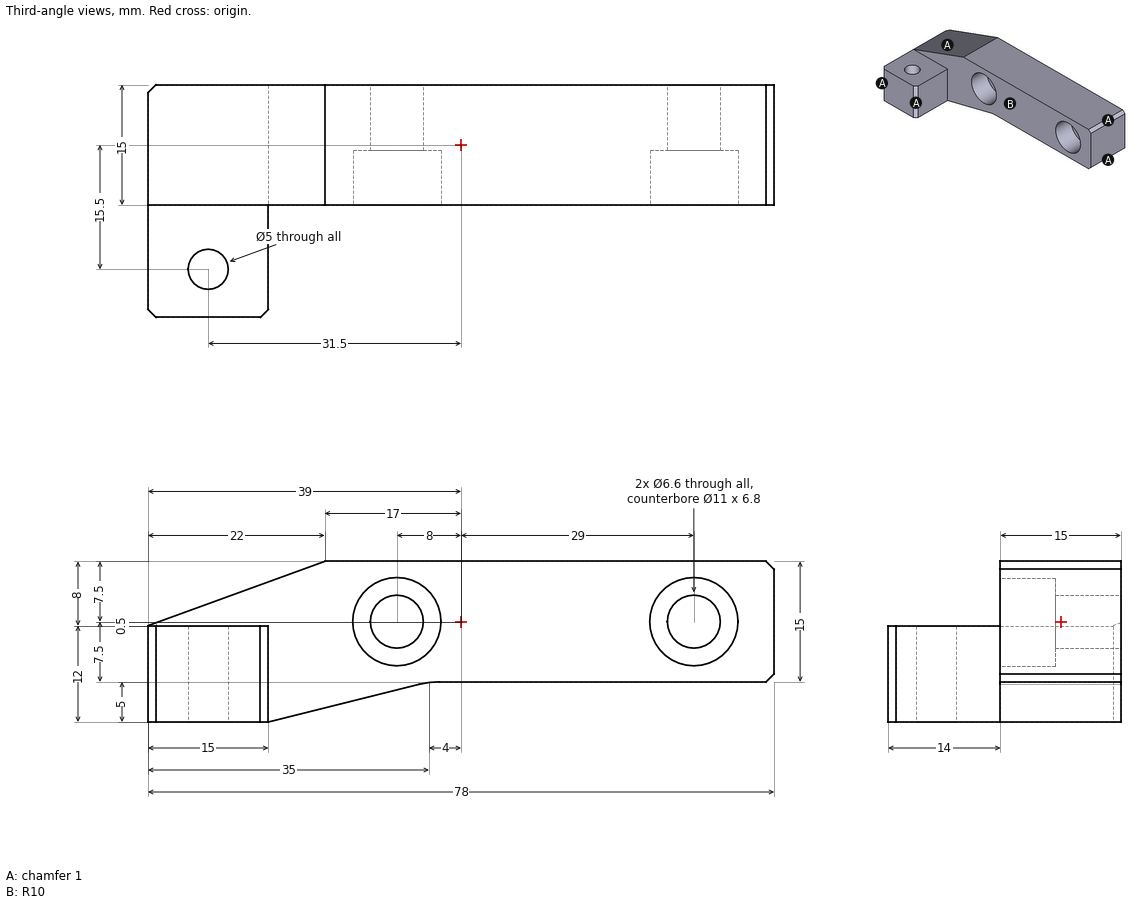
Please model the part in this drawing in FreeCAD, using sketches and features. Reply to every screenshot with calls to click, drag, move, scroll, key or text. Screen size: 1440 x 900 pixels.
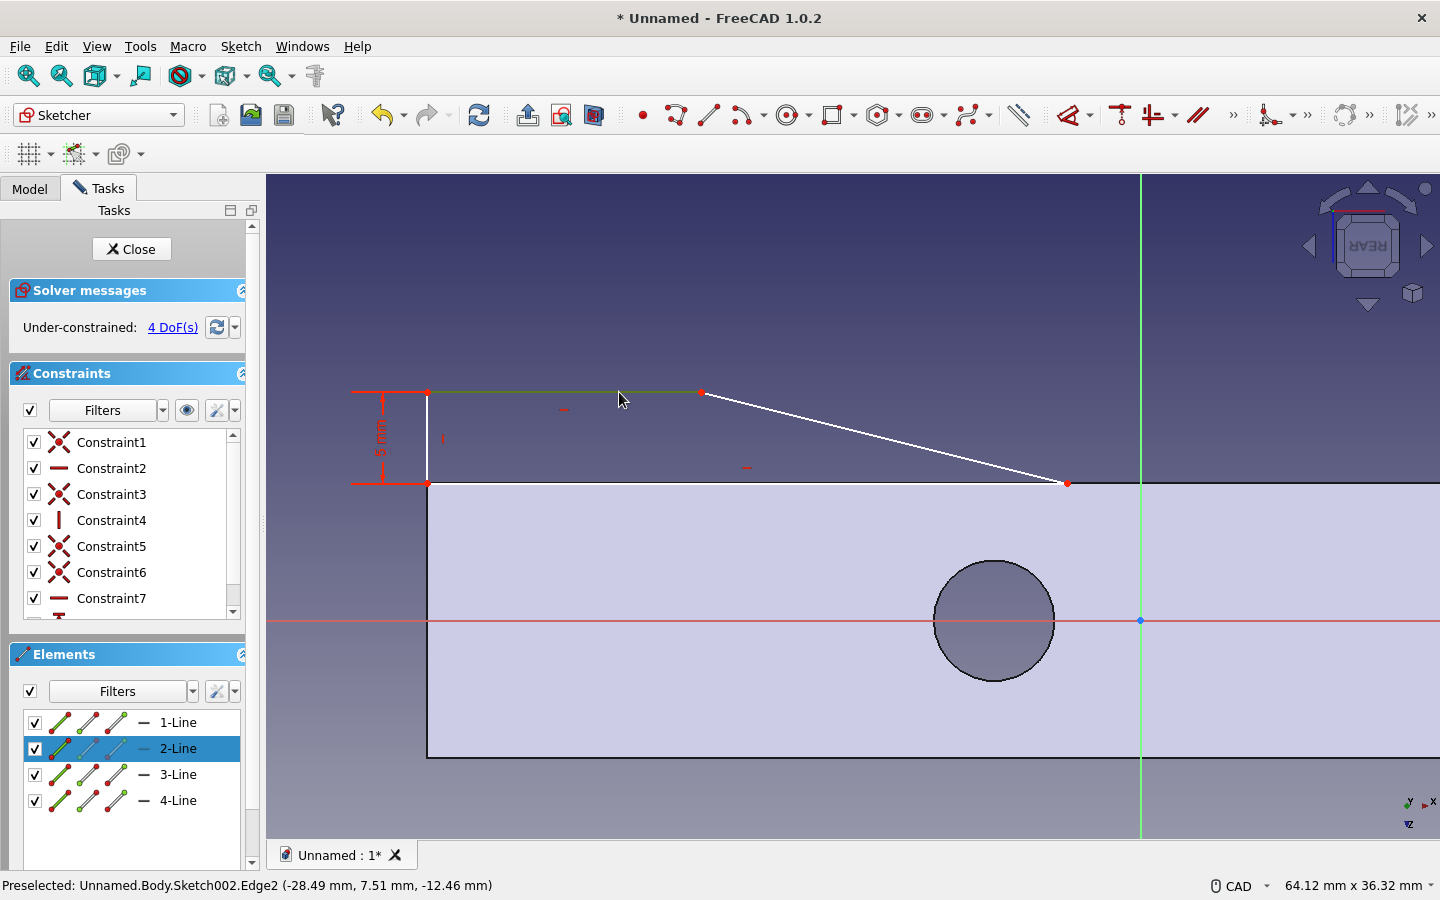
key(l)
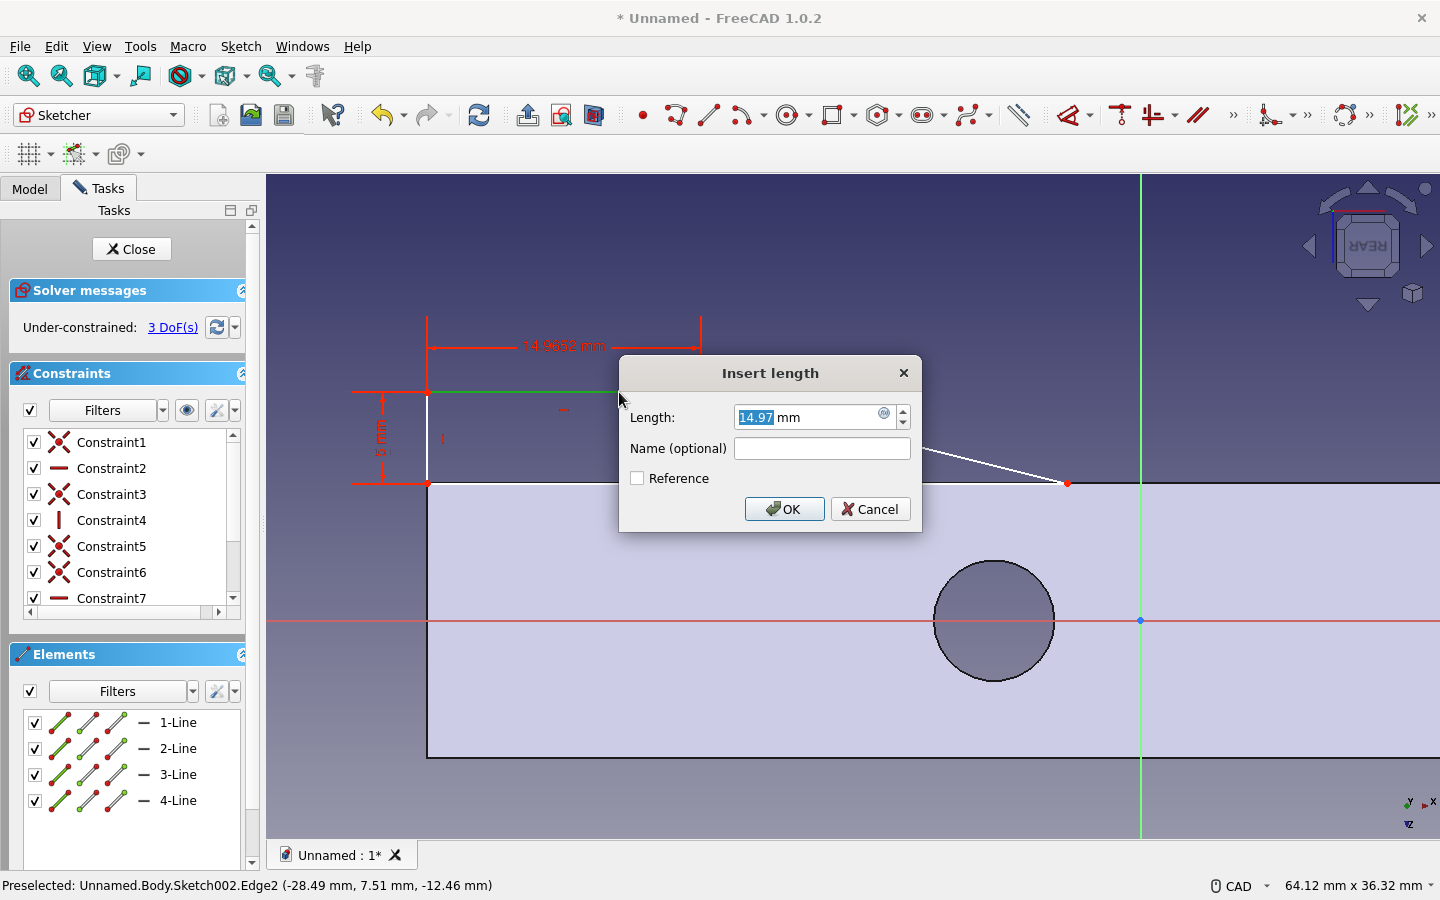
text(15)
key(Return)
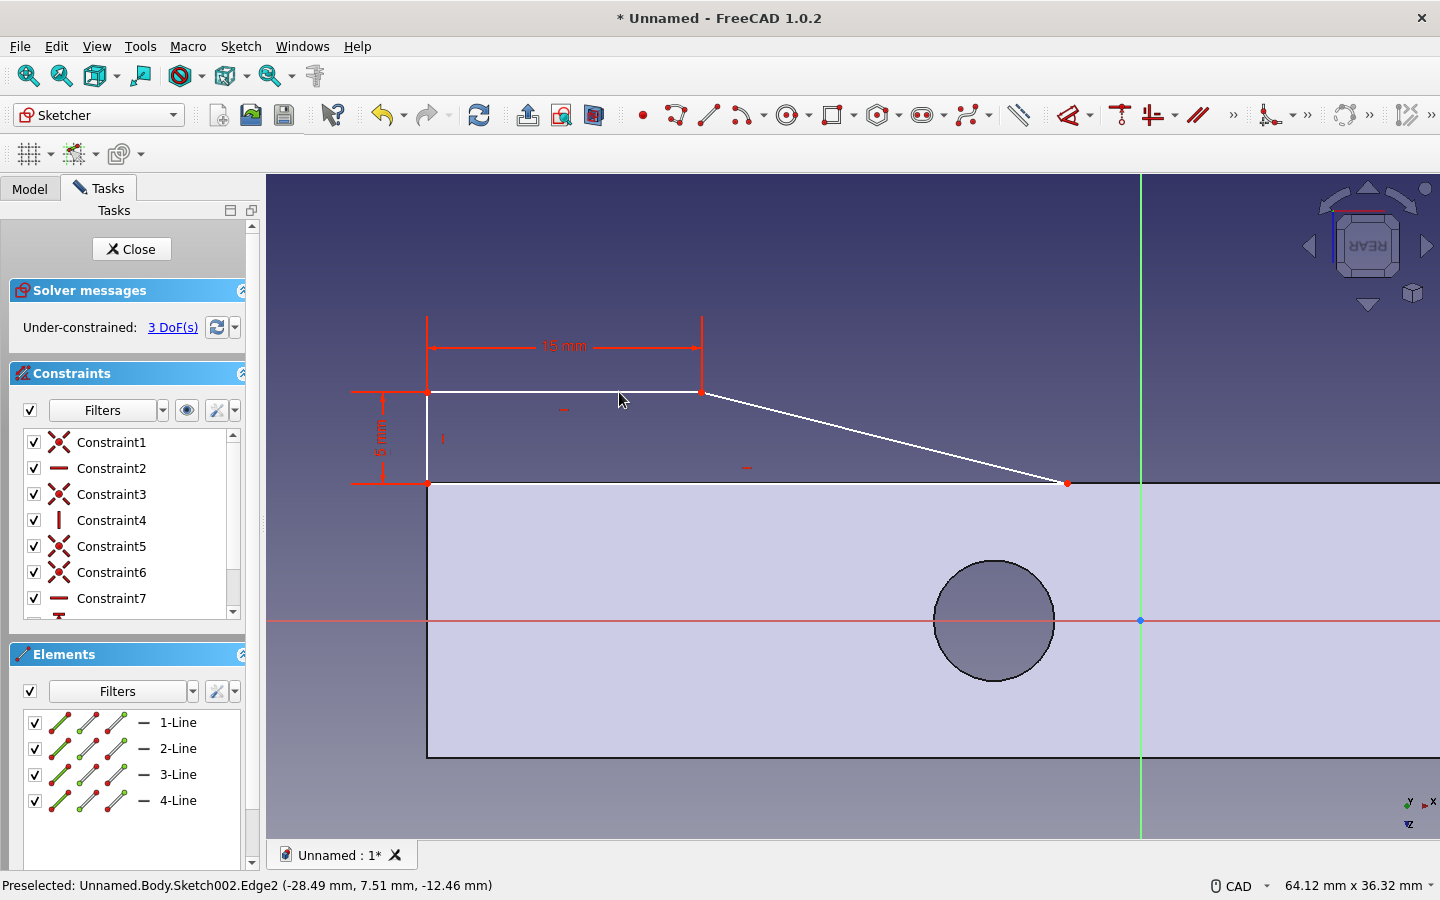
click(619, 484)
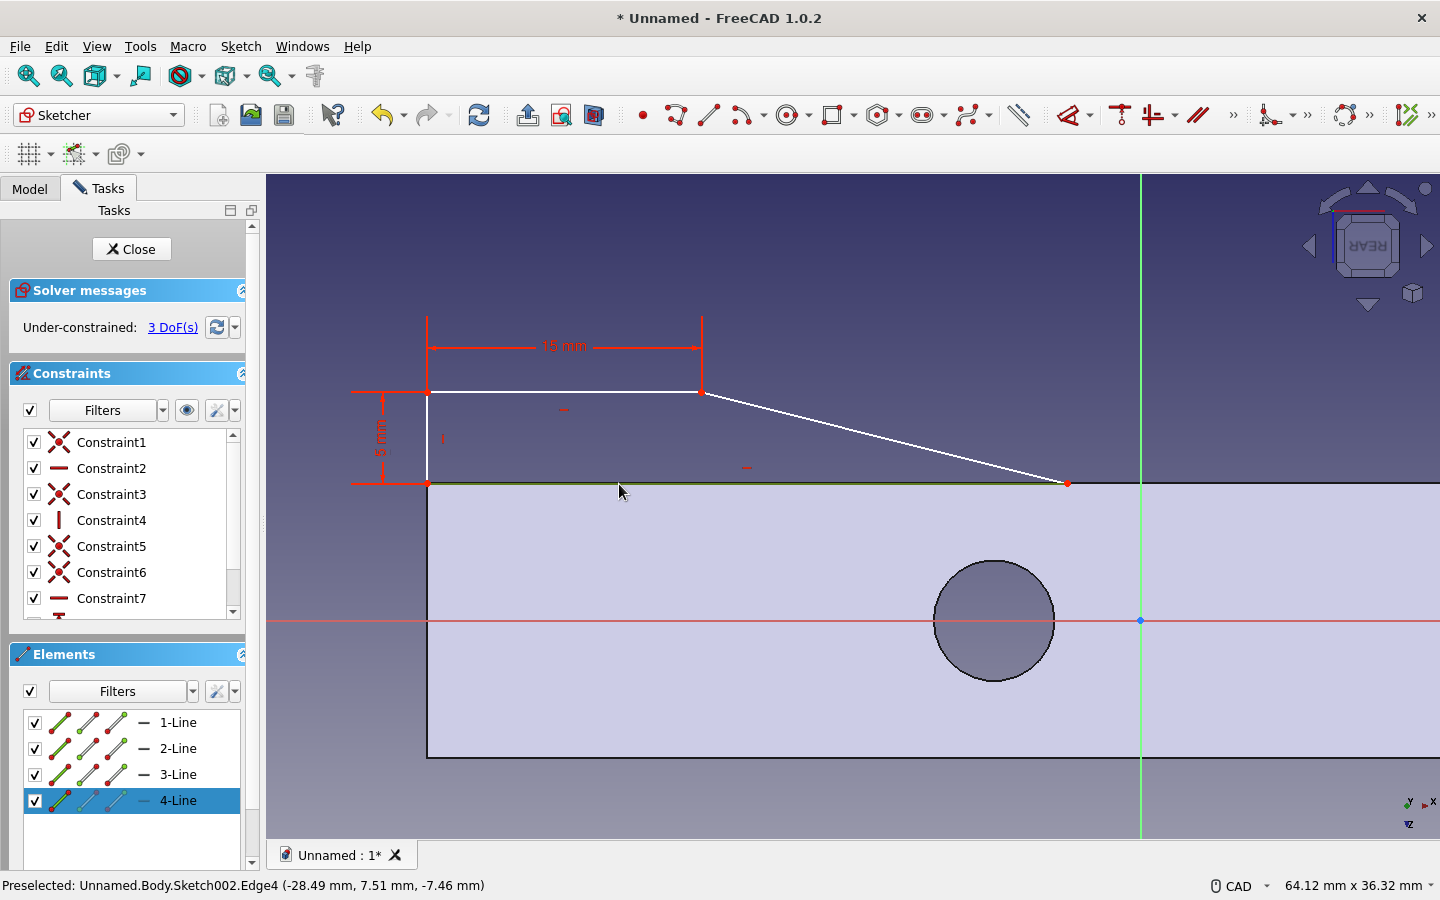
key(l)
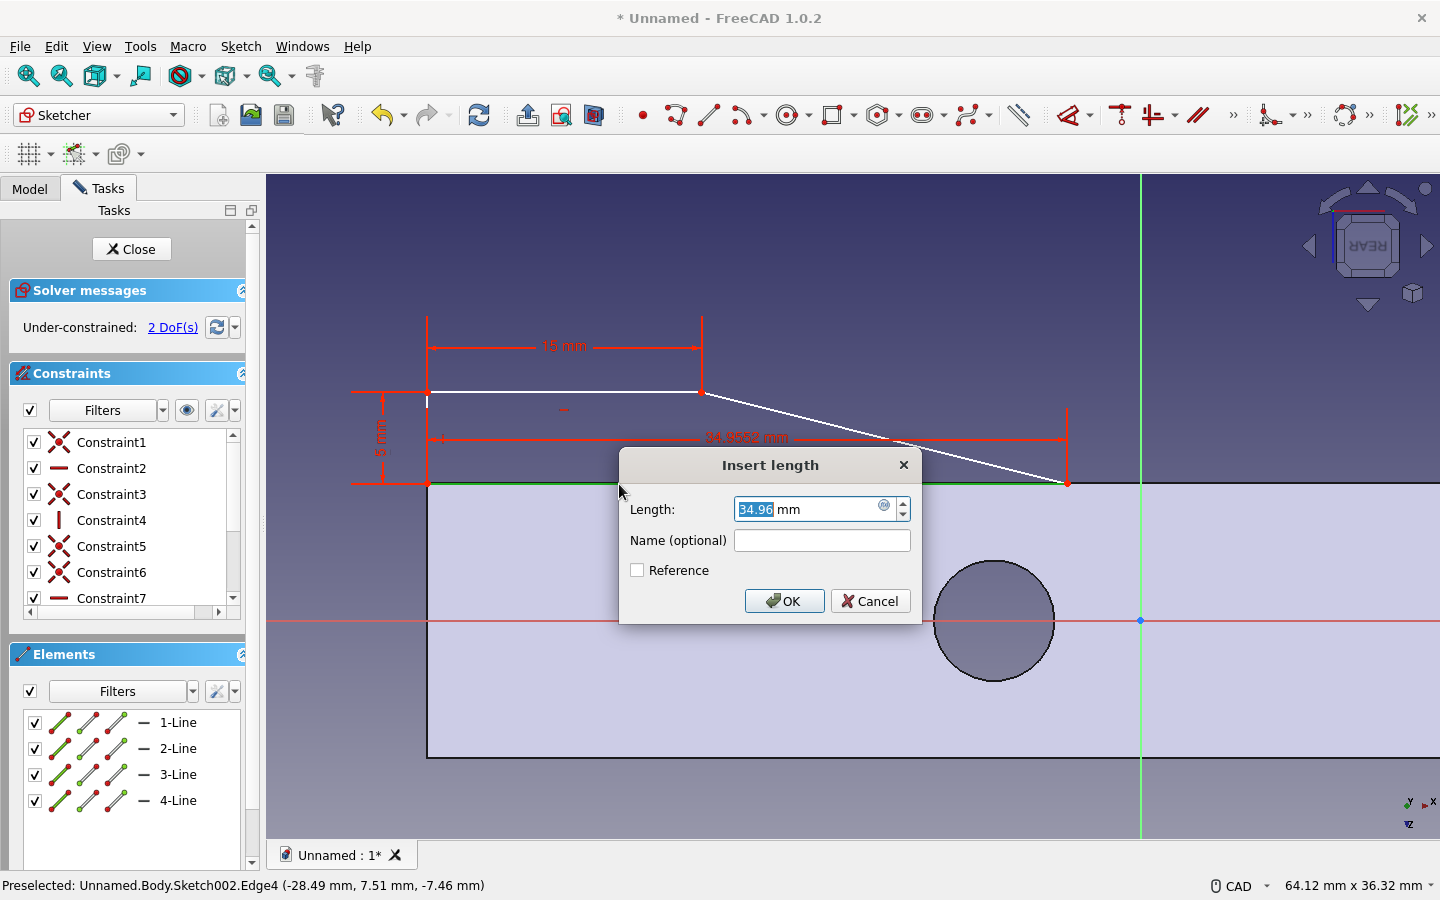
text(35)
key(Return)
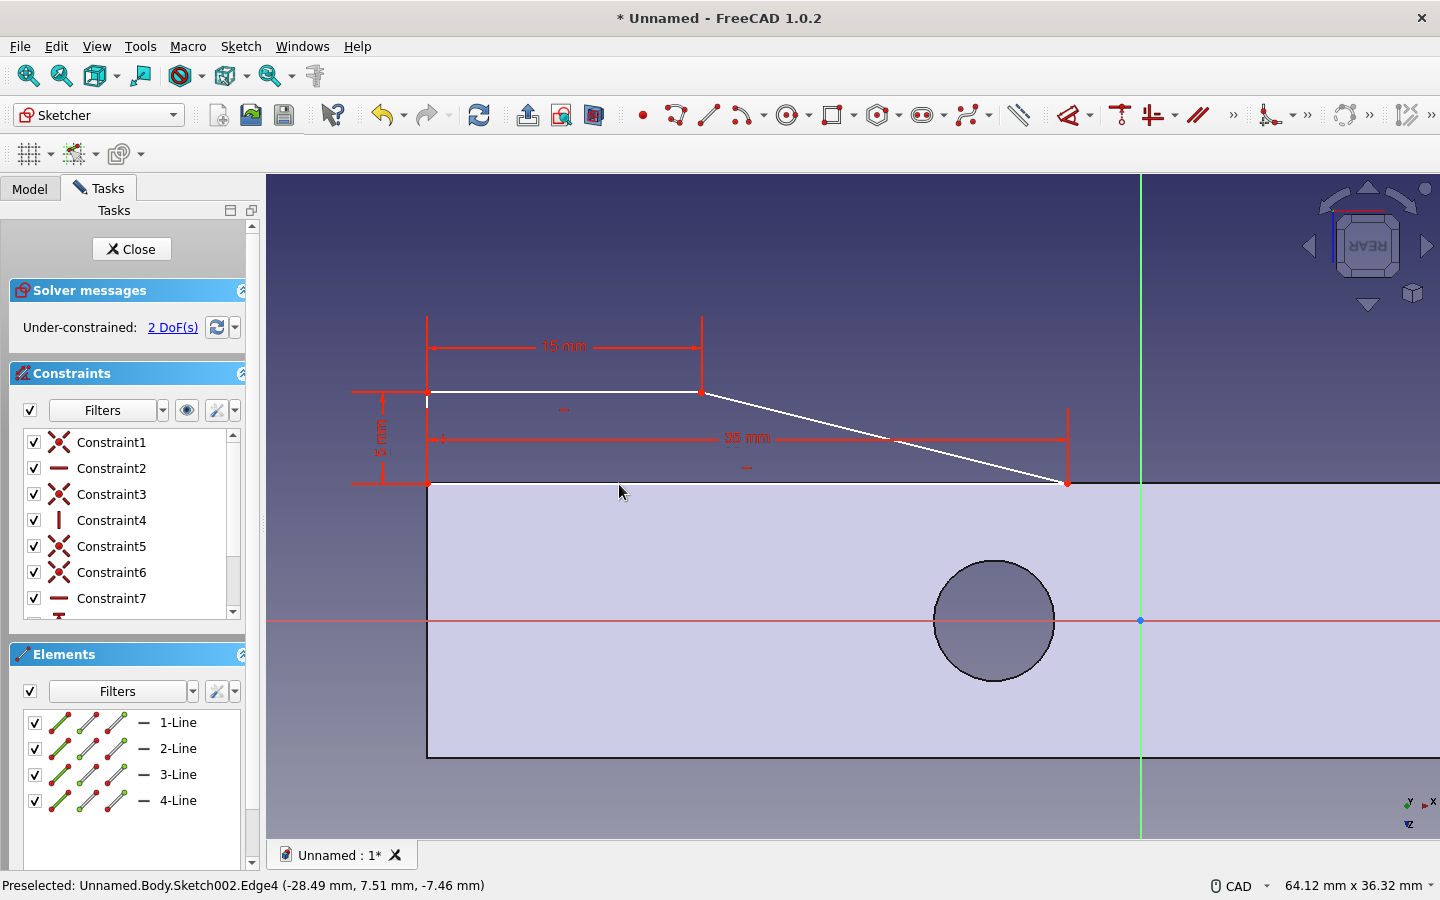
click(1068, 484)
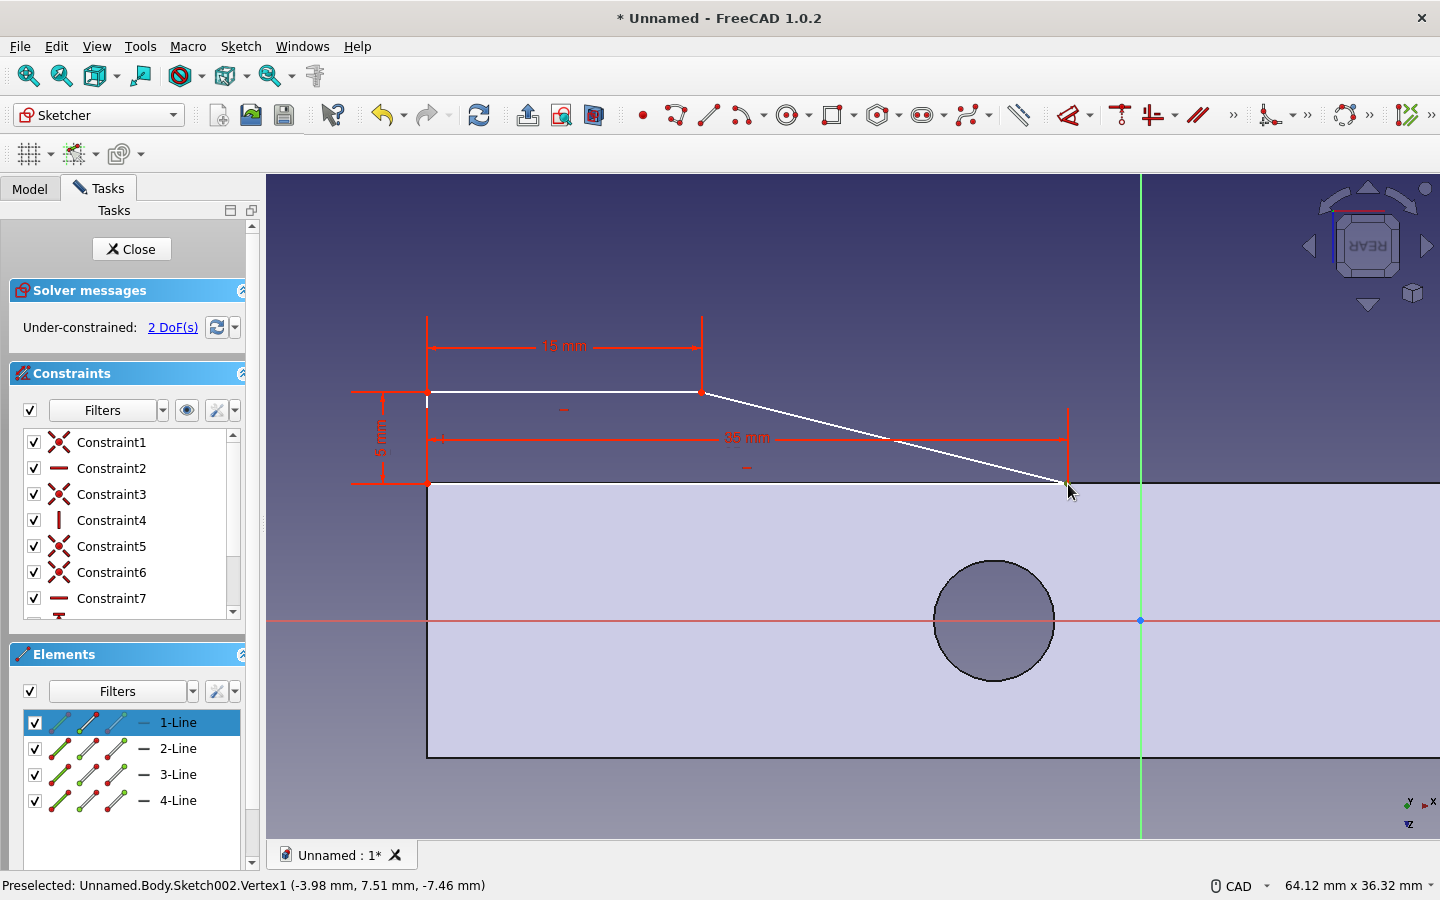
click(1090, 116)